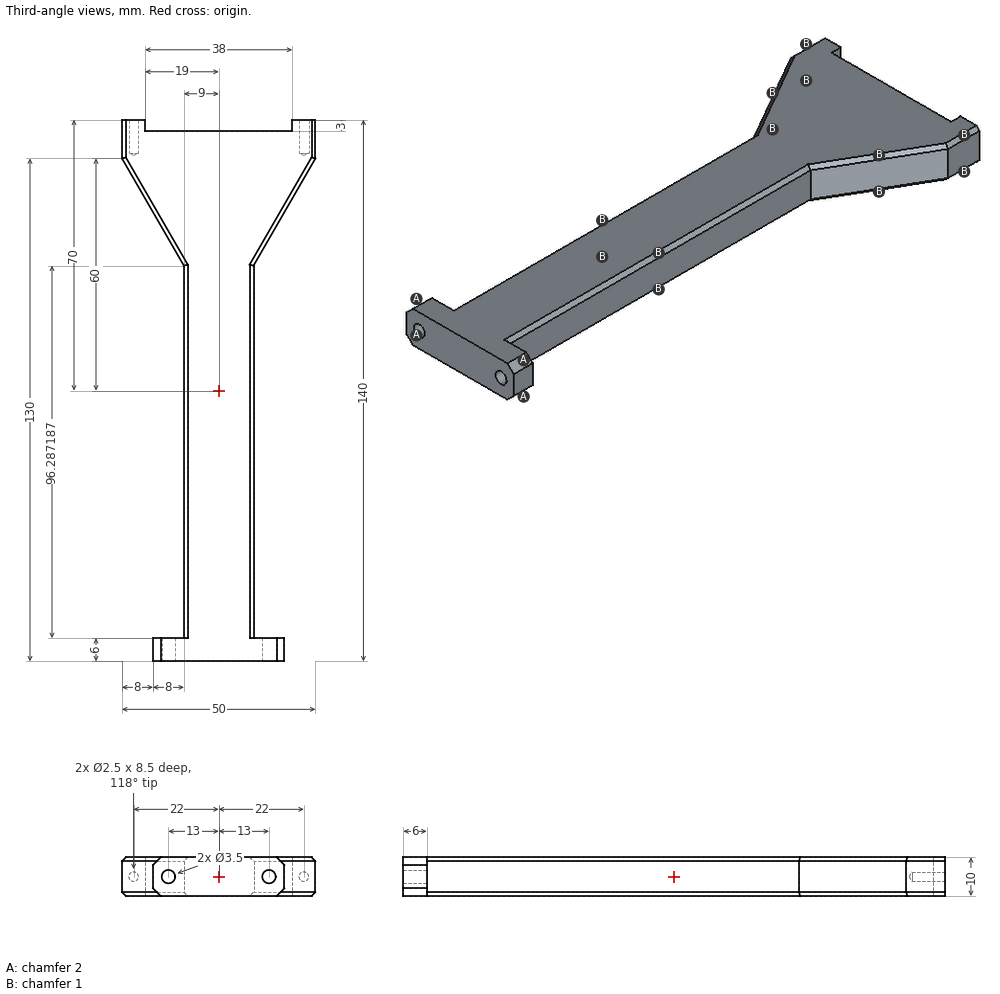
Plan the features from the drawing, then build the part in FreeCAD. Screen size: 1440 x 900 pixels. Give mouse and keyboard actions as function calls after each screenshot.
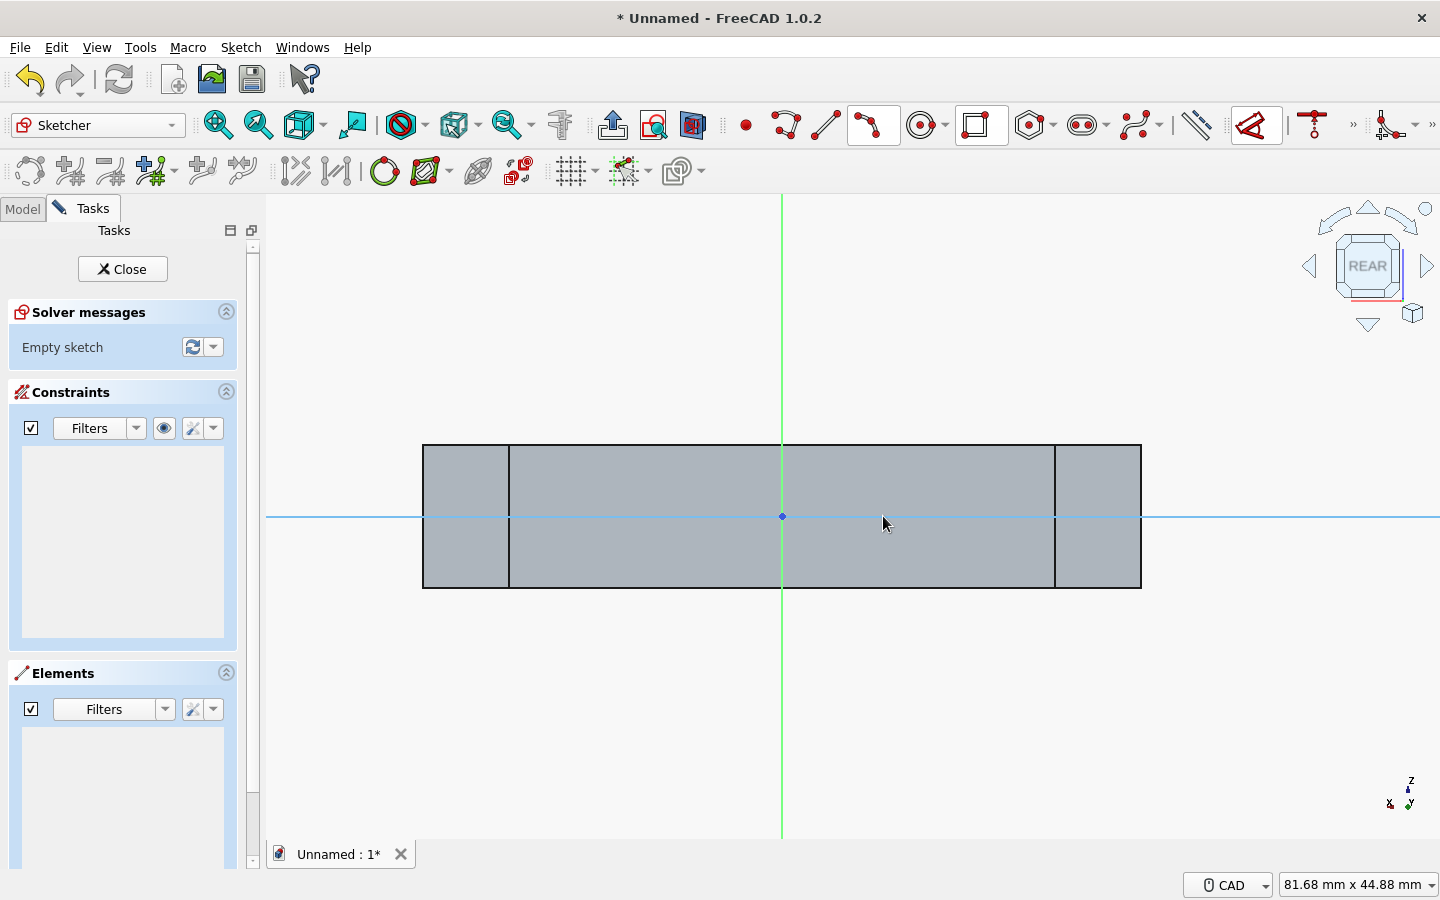
click(922, 126)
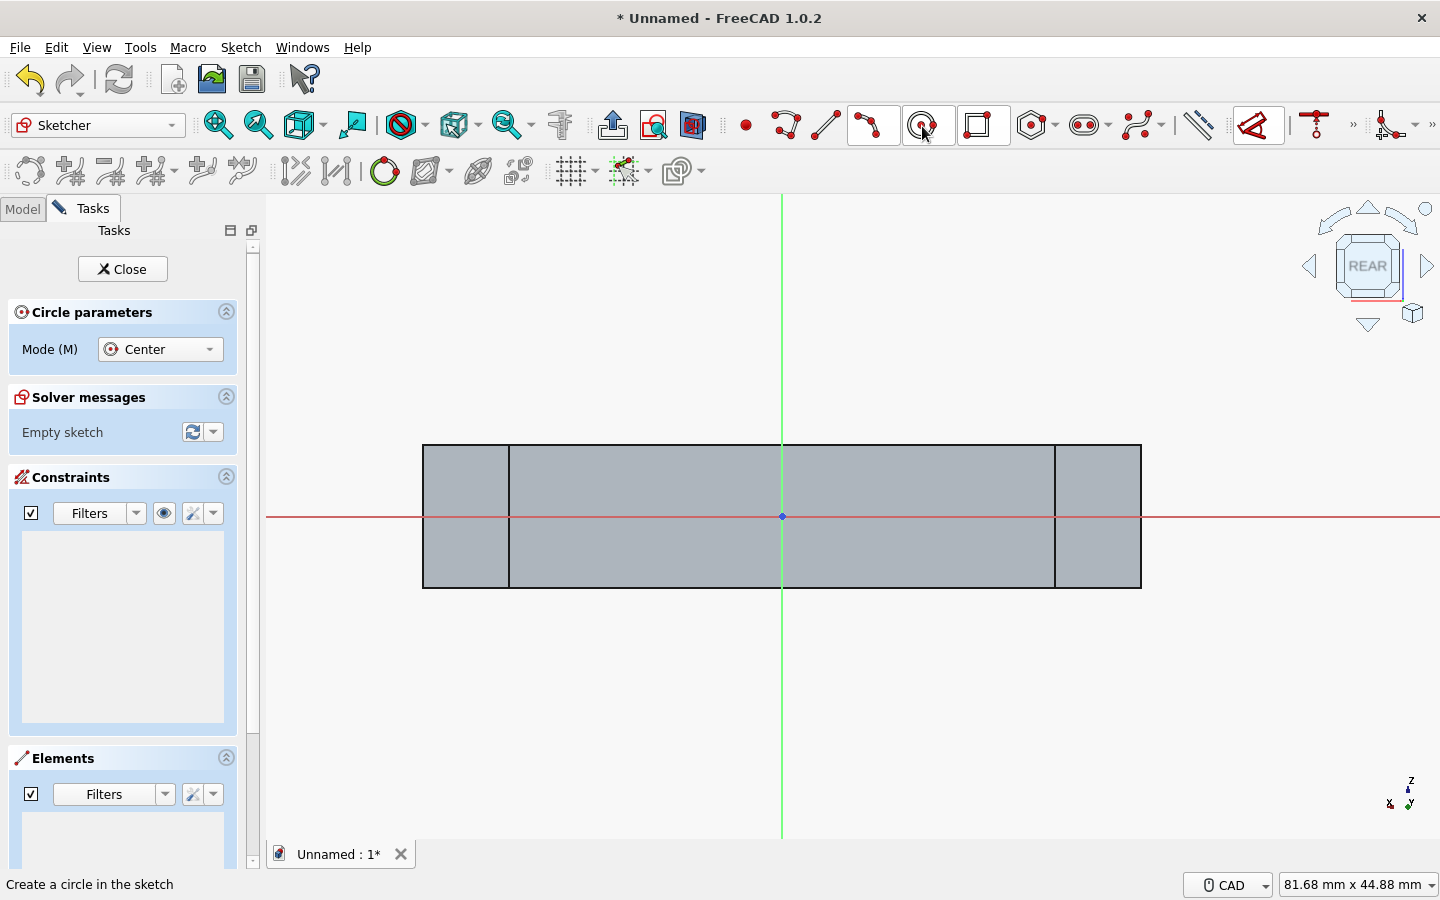
scroll(1098, 516, up, 2)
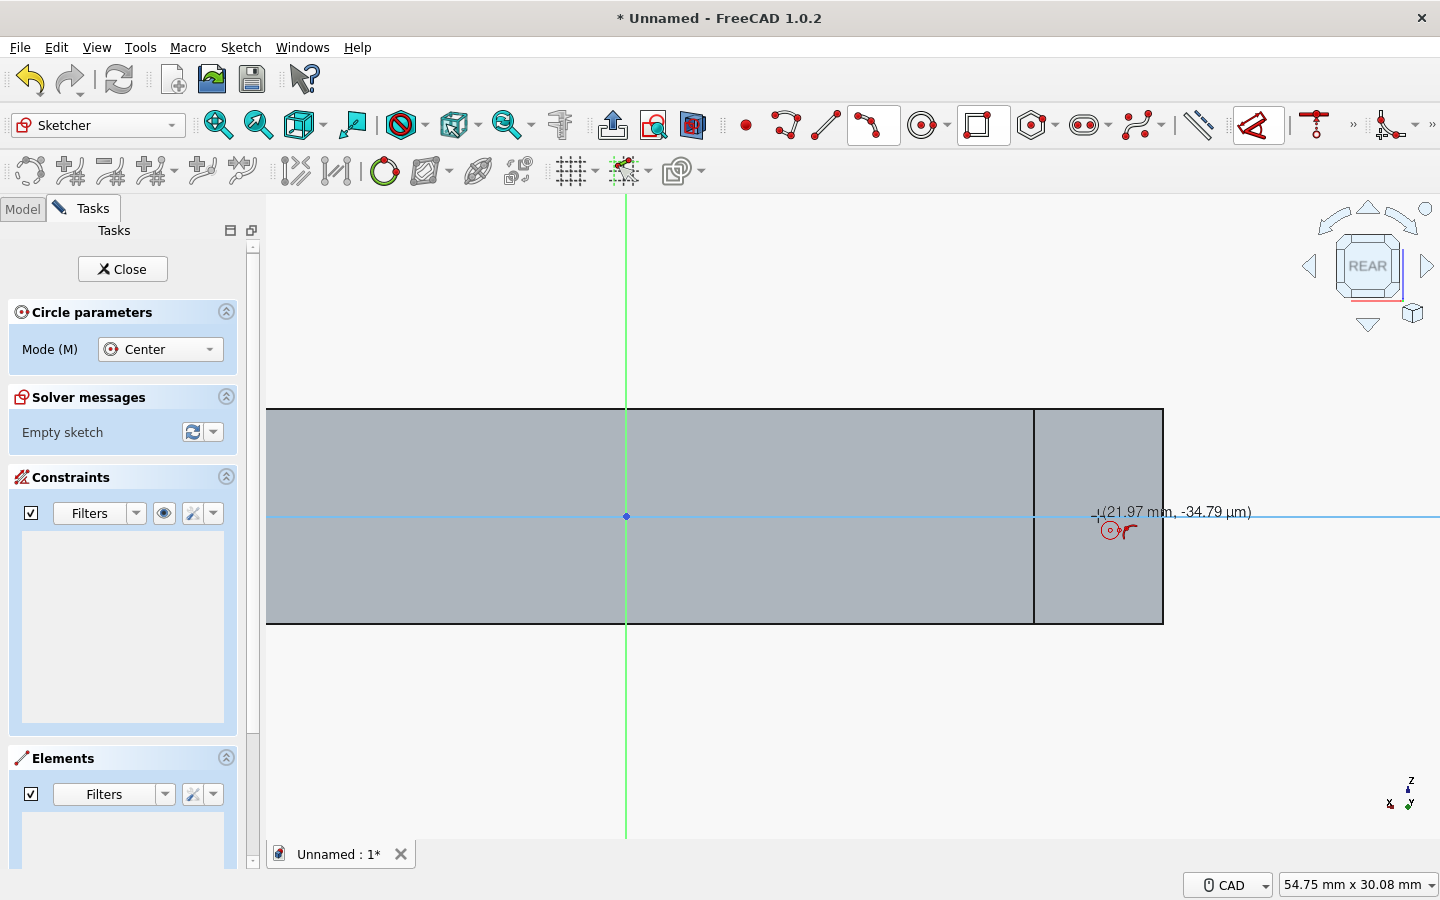
click(1098, 516)
move(1117, 498)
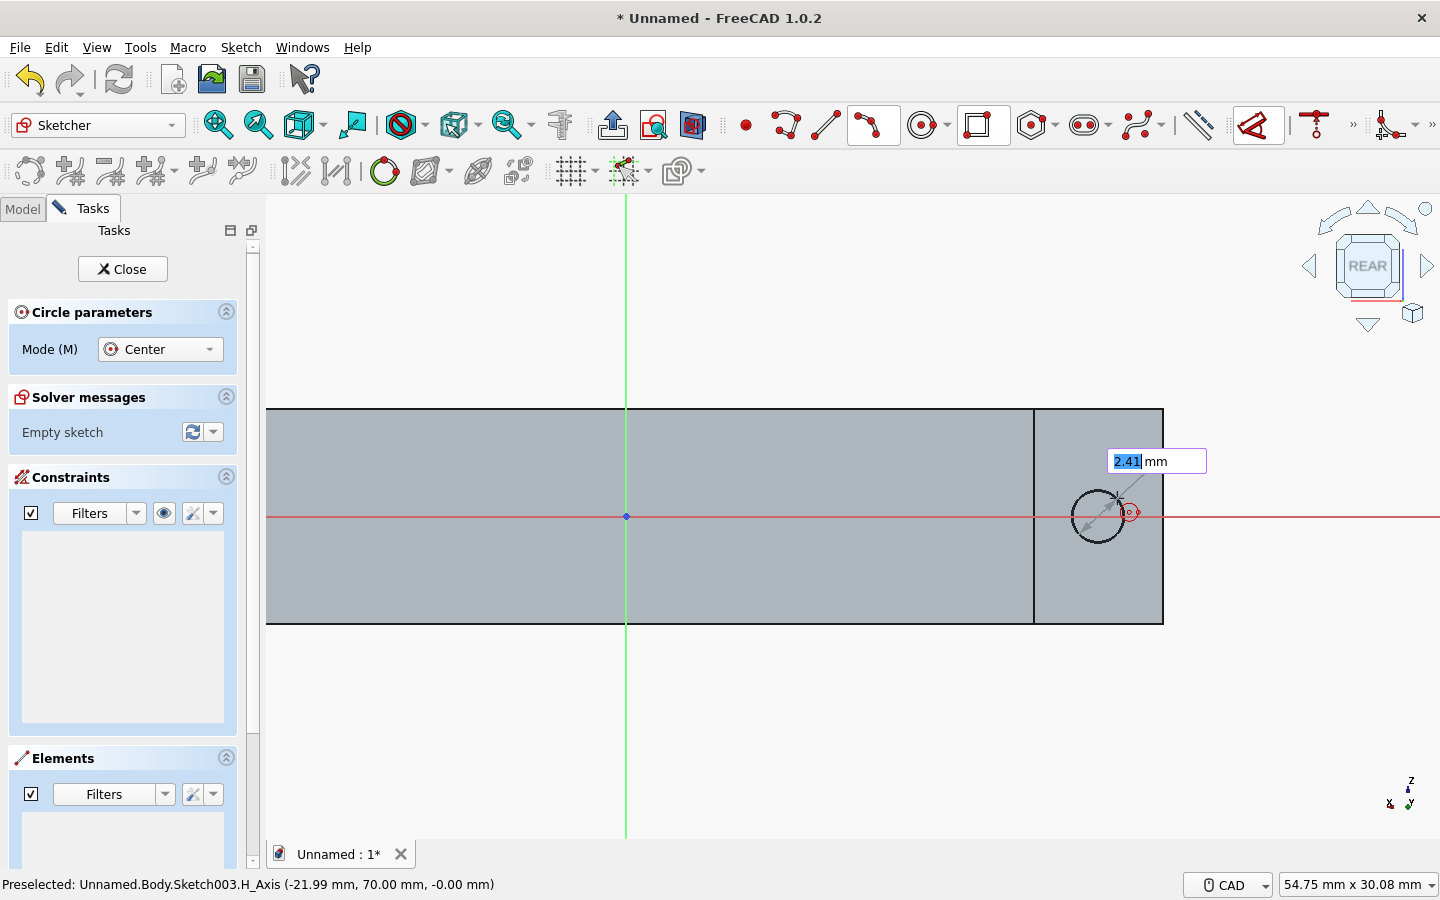
text(2.5)
key(Return)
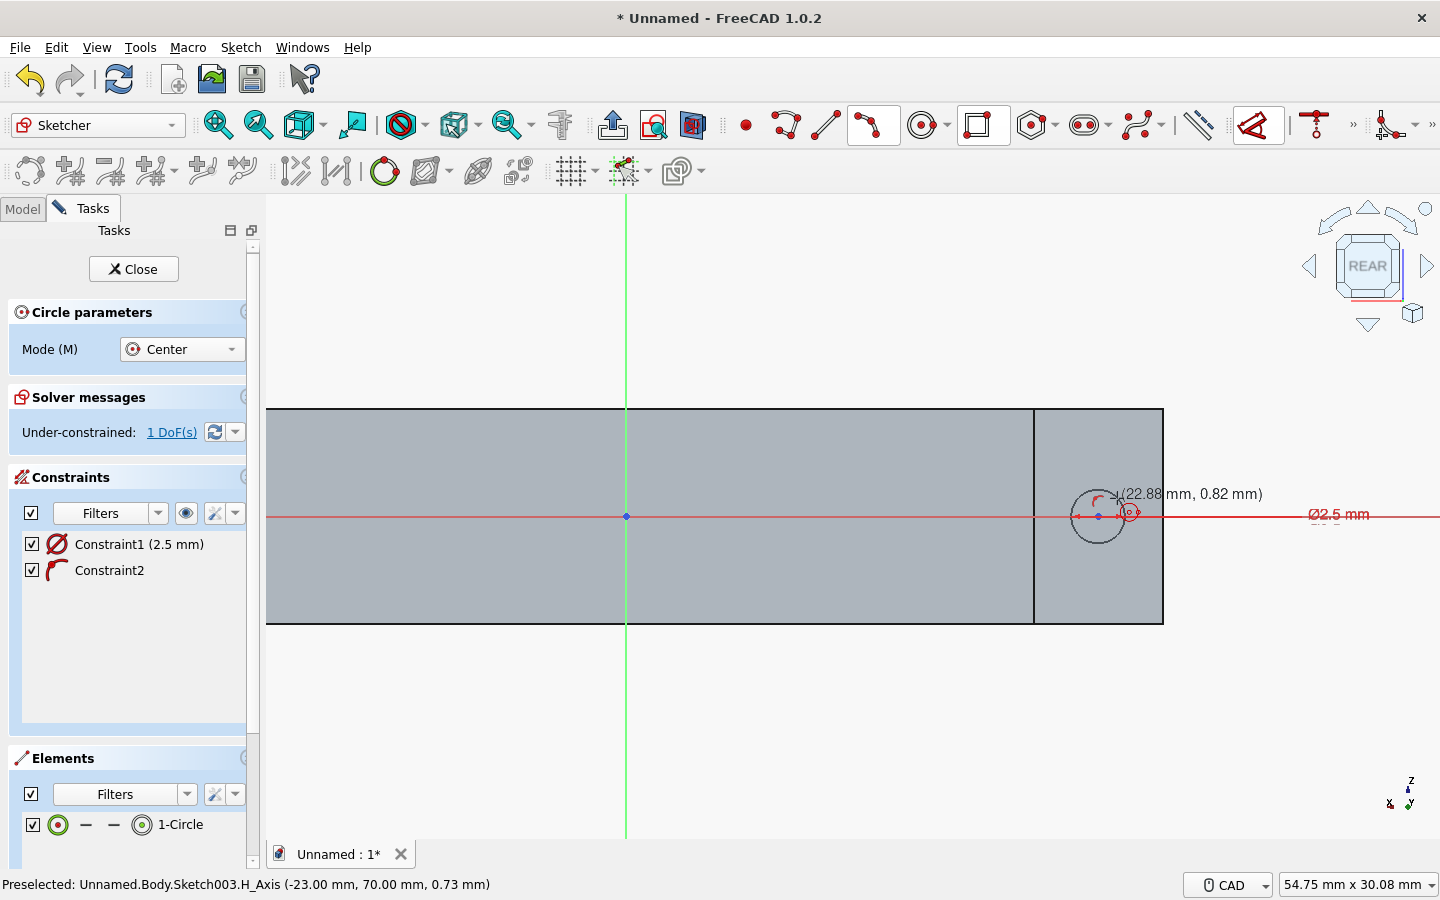
scroll(1106, 516, down, 2)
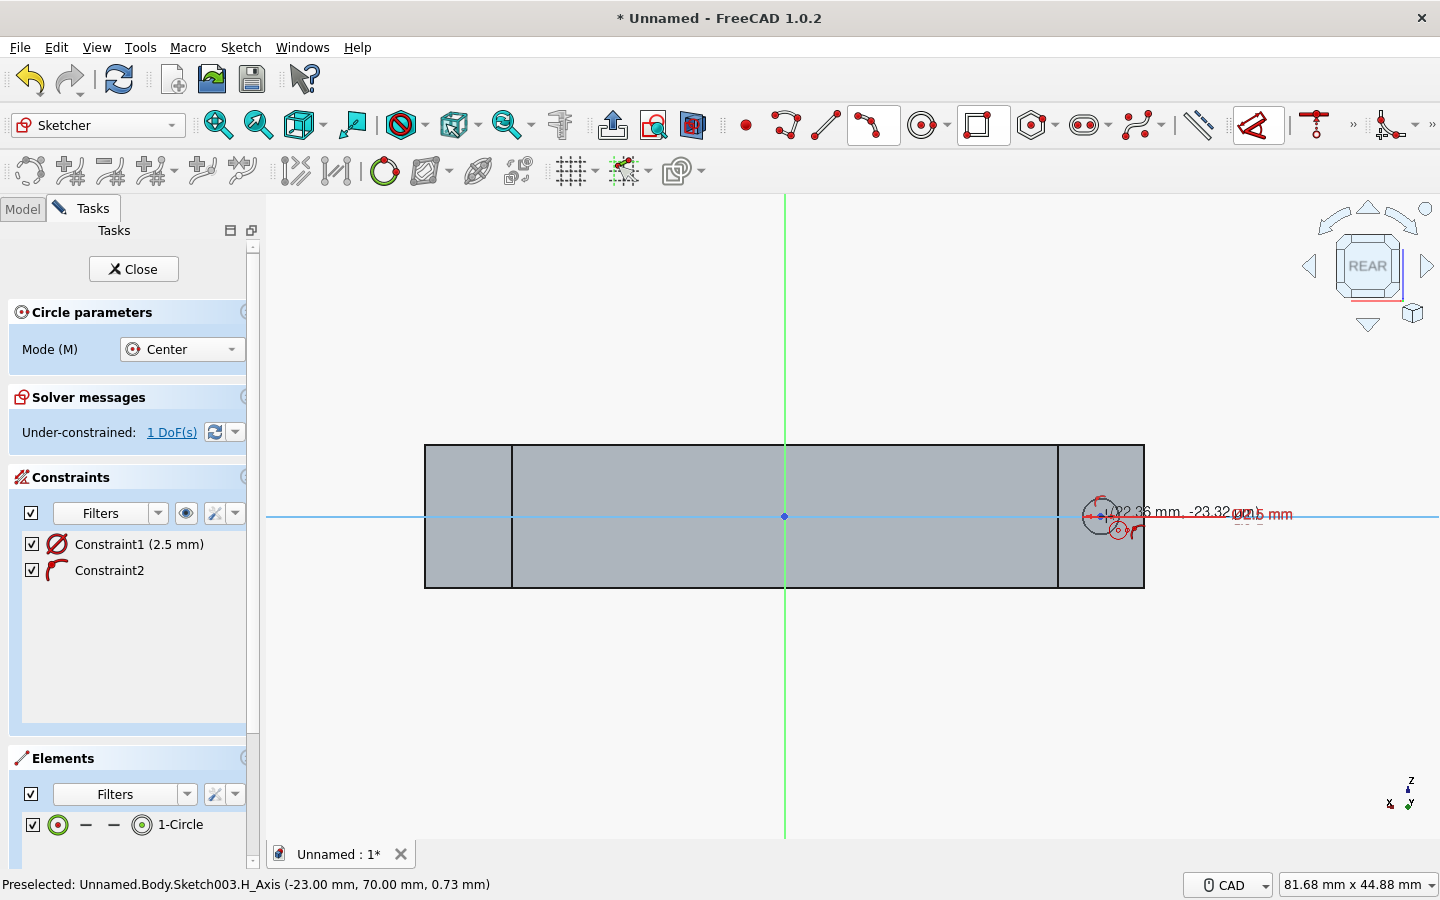
scroll(469, 516, up, 2)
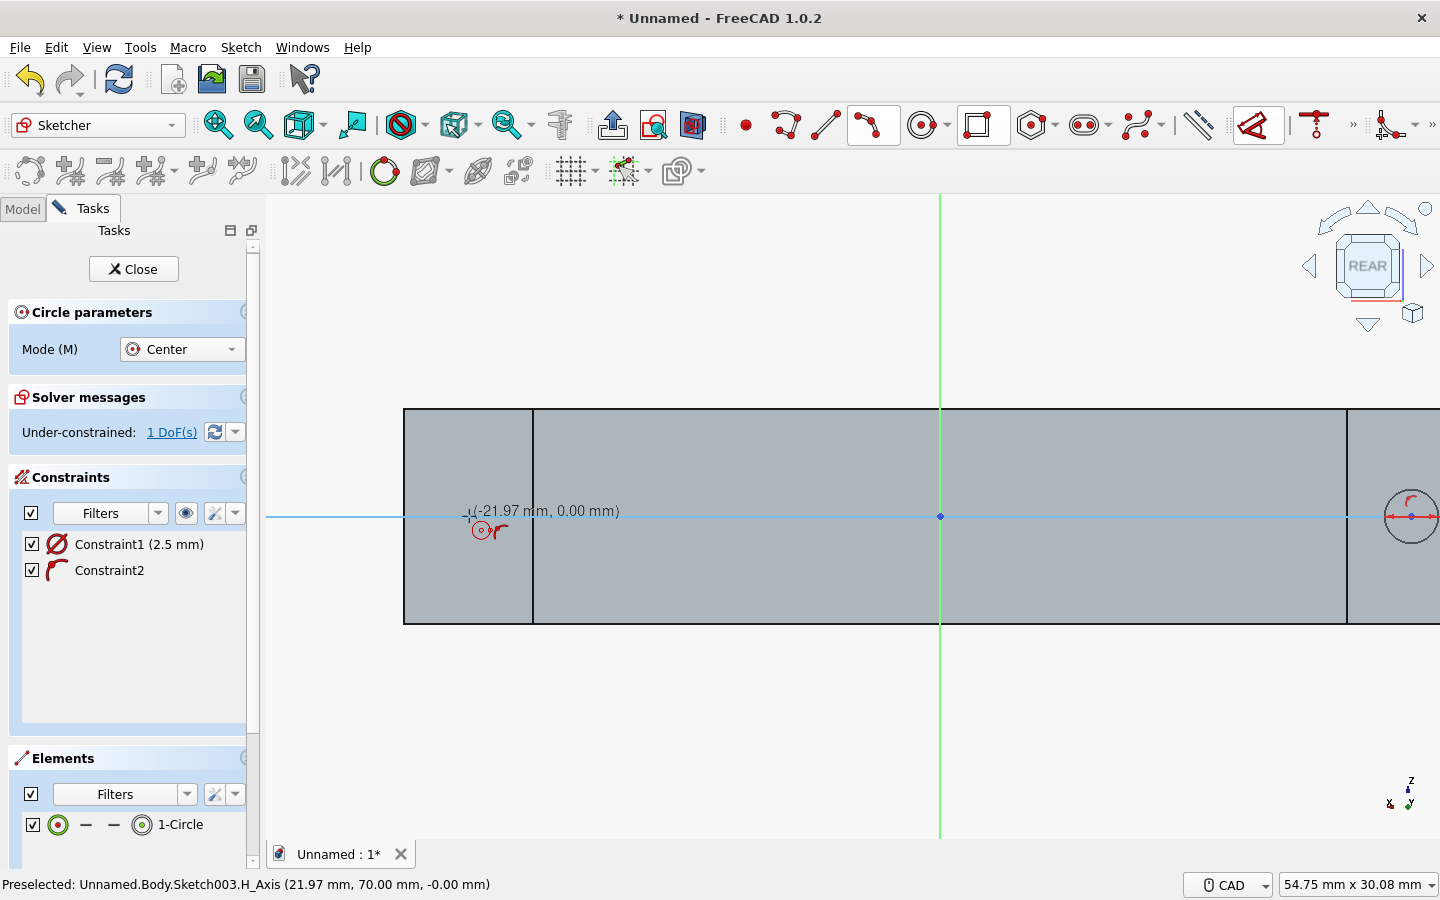
click(468, 516)
move(487, 498)